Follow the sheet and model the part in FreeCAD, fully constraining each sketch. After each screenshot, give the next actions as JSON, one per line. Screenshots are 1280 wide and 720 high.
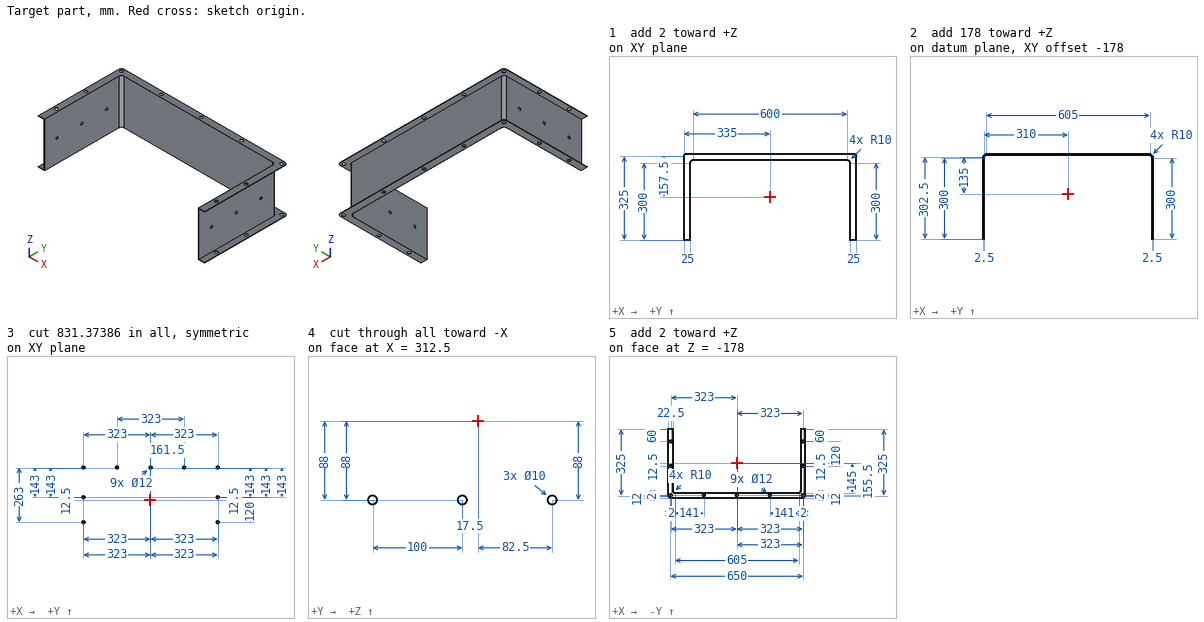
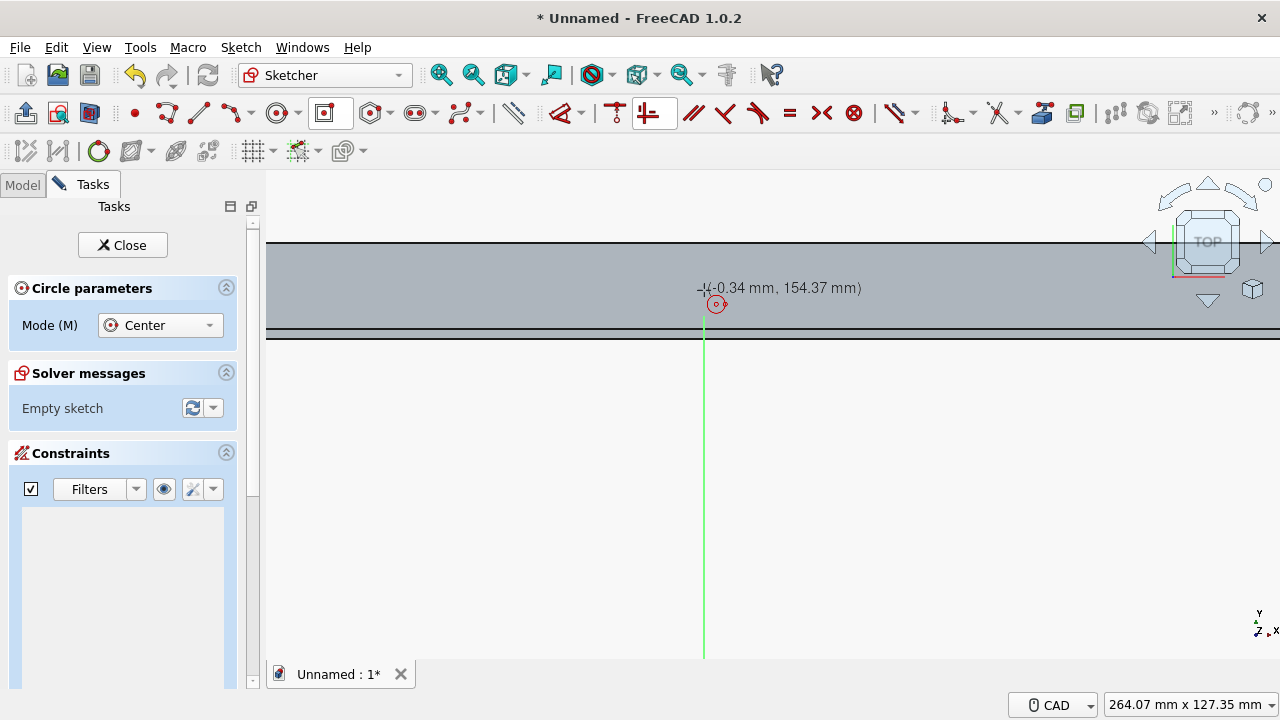
{"action": "scroll", "coordinate": [705, 290], "scroll_direction": "down", "scroll_amount": 7}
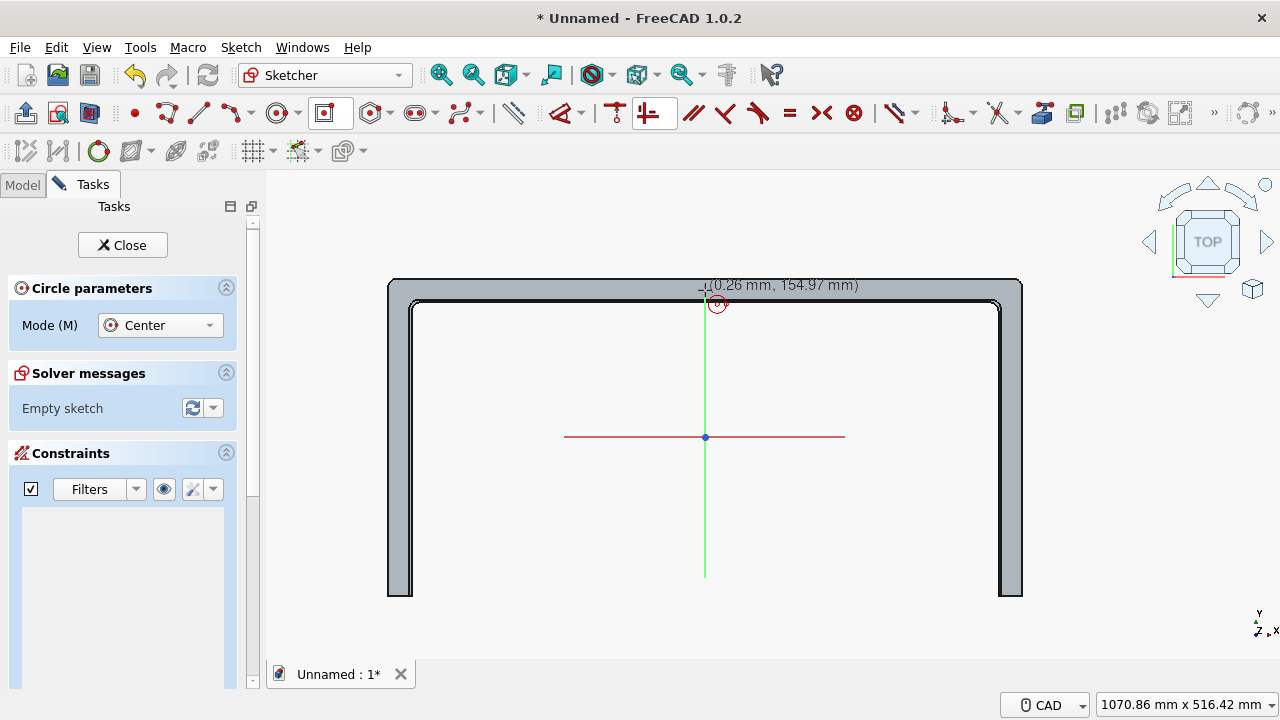
{"action": "left_click", "coordinate": [705, 290]}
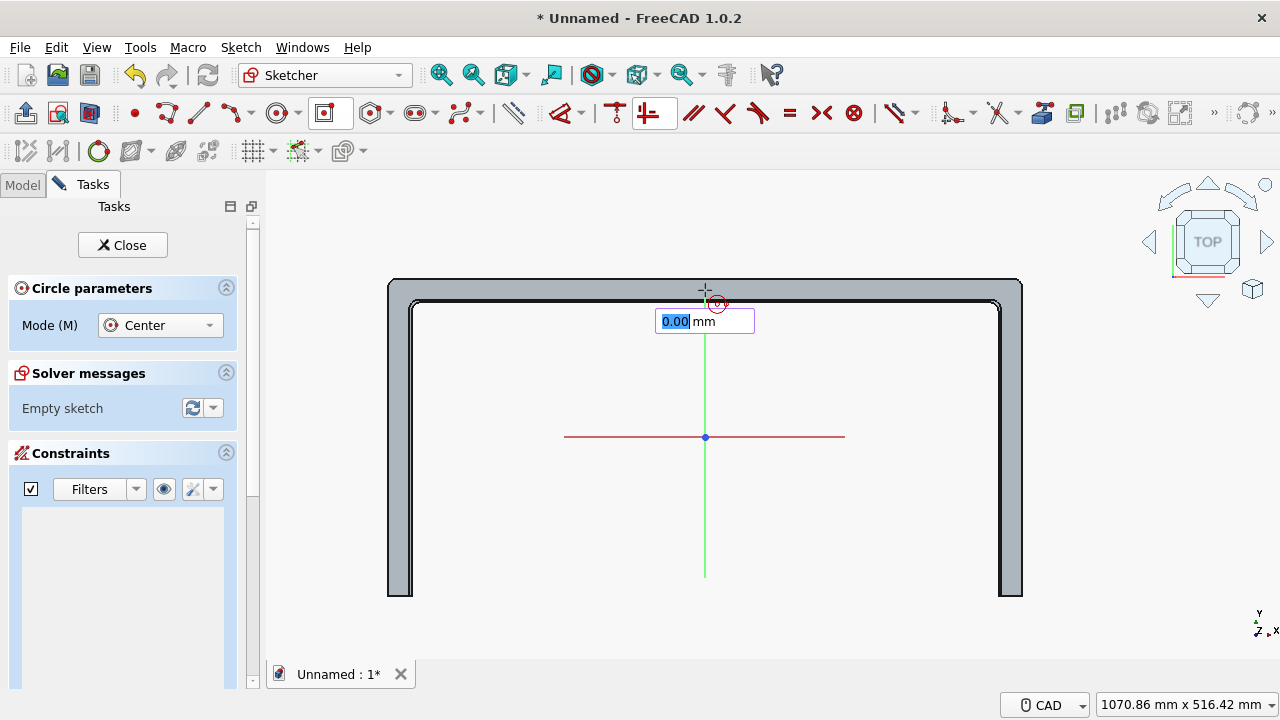
{"action": "scroll", "coordinate": [710, 288], "scroll_direction": "up", "scroll_amount": 6}
{"action": "mouse_move", "coordinate": [710, 287]}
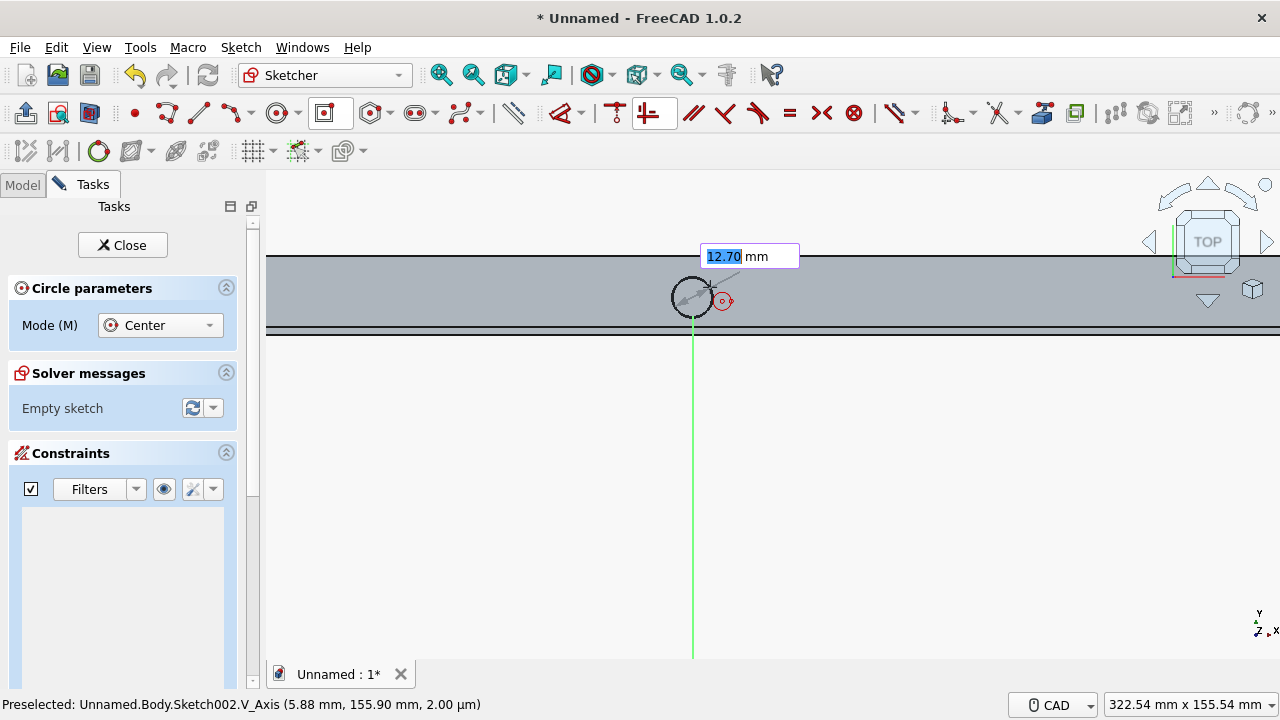
{"action": "type", "text": "12"}
{"action": "key", "text": "Return"}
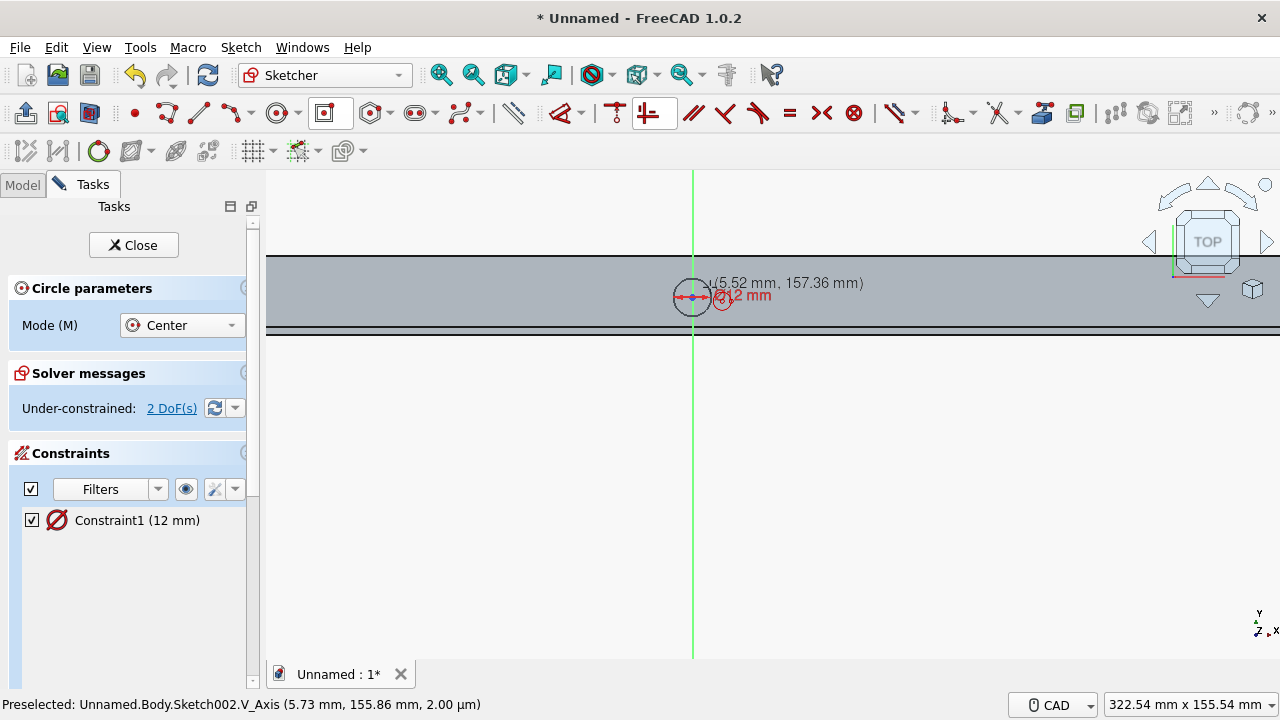
{"action": "scroll", "coordinate": [710, 288], "scroll_direction": "down", "scroll_amount": 6}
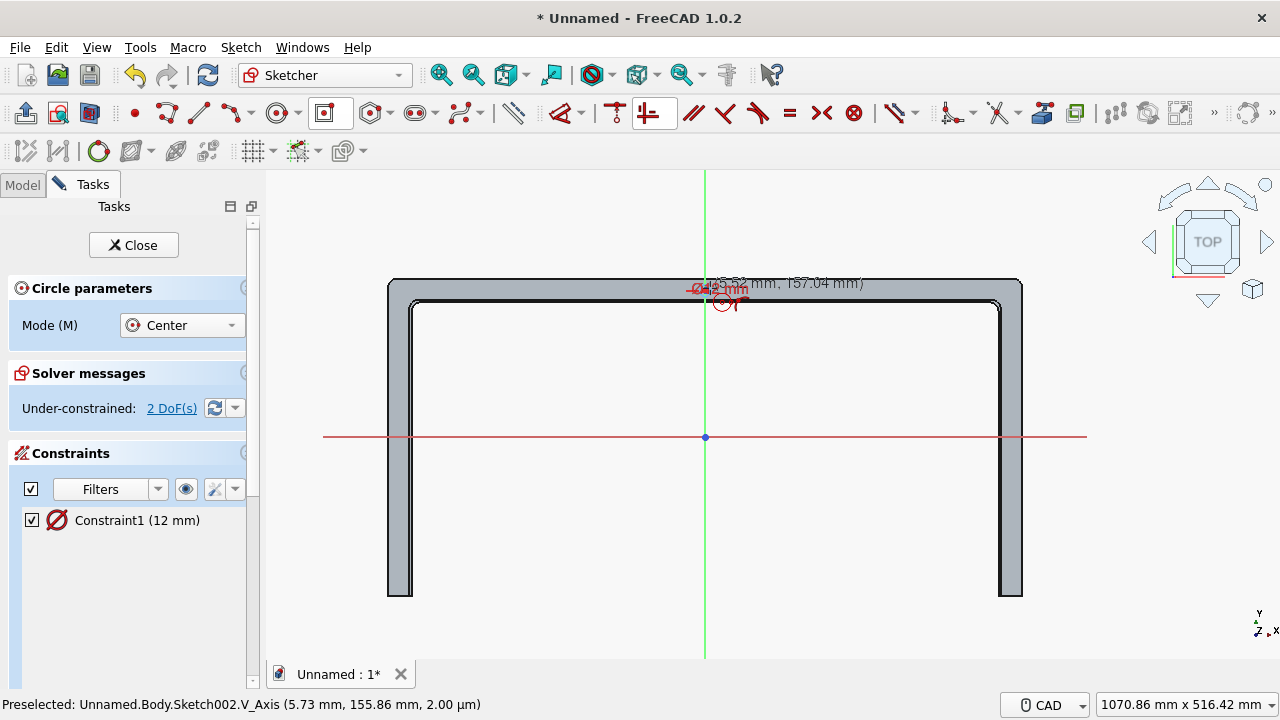
{"action": "scroll", "coordinate": [858, 290], "scroll_direction": "up", "scroll_amount": 7}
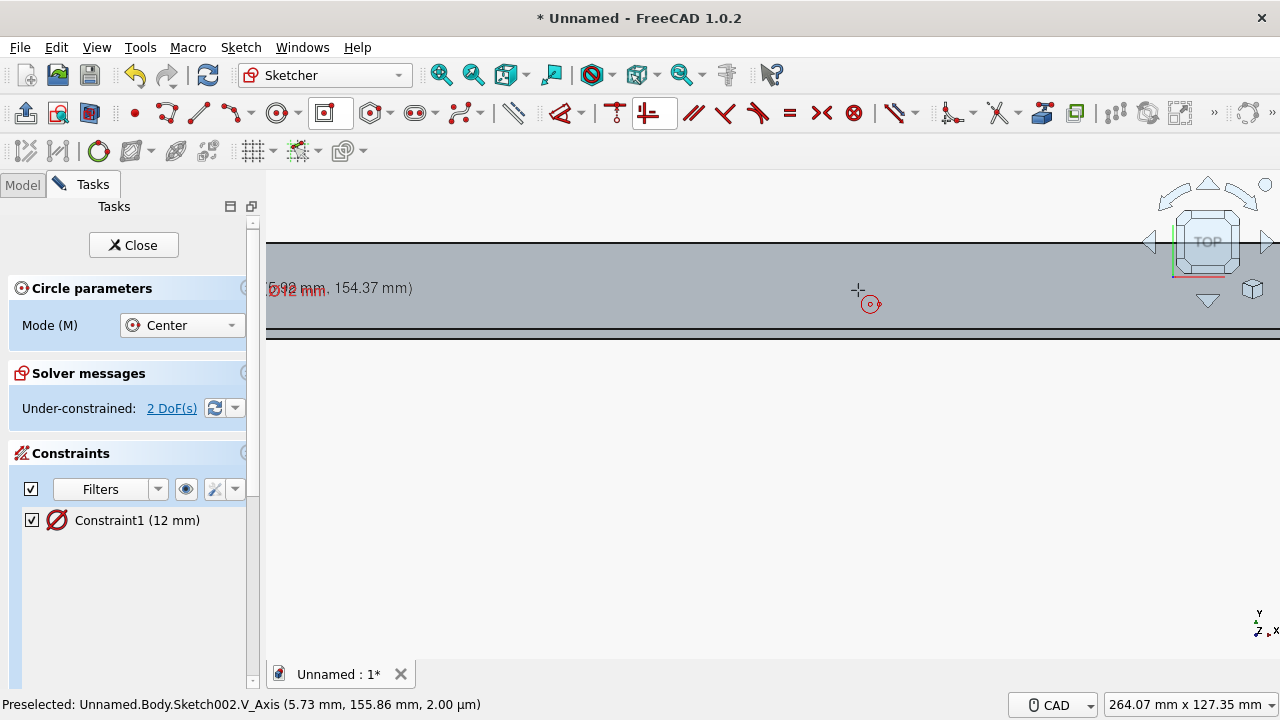
{"action": "scroll", "coordinate": [858, 290], "scroll_direction": "down", "scroll_amount": 7}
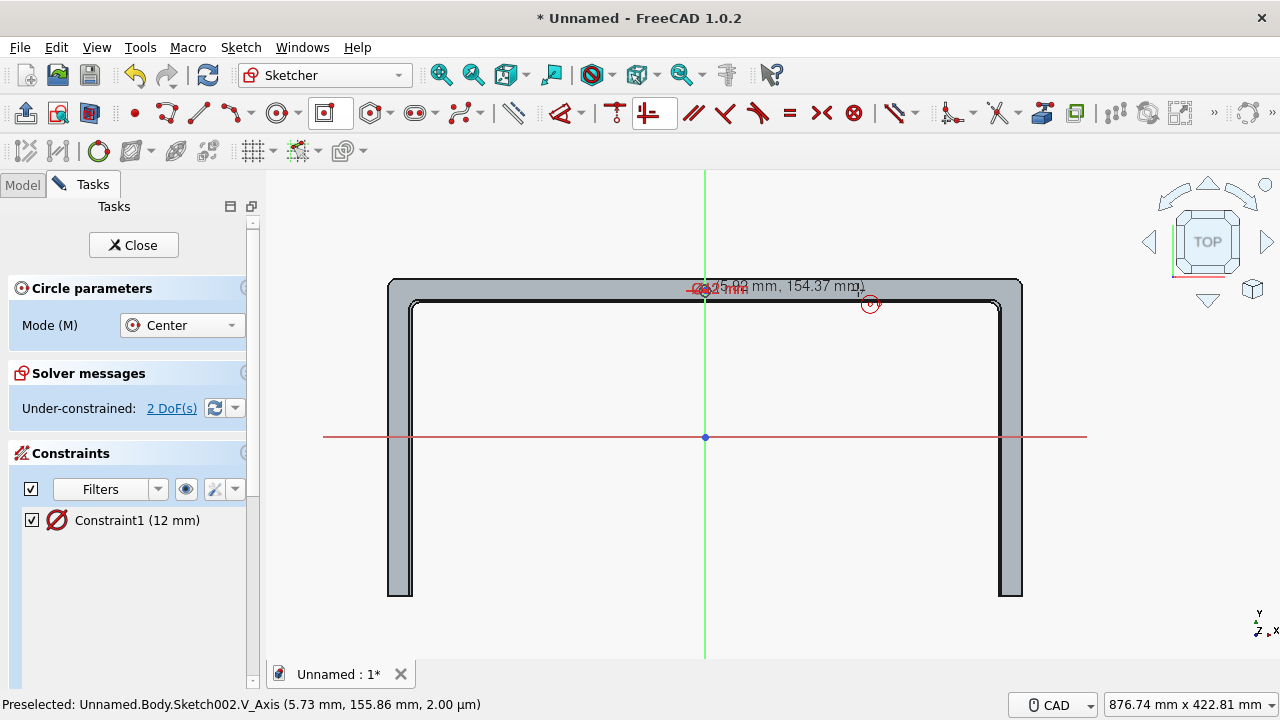
{"action": "left_click", "coordinate": [858, 290]}
{"action": "mouse_move", "coordinate": [862, 286]}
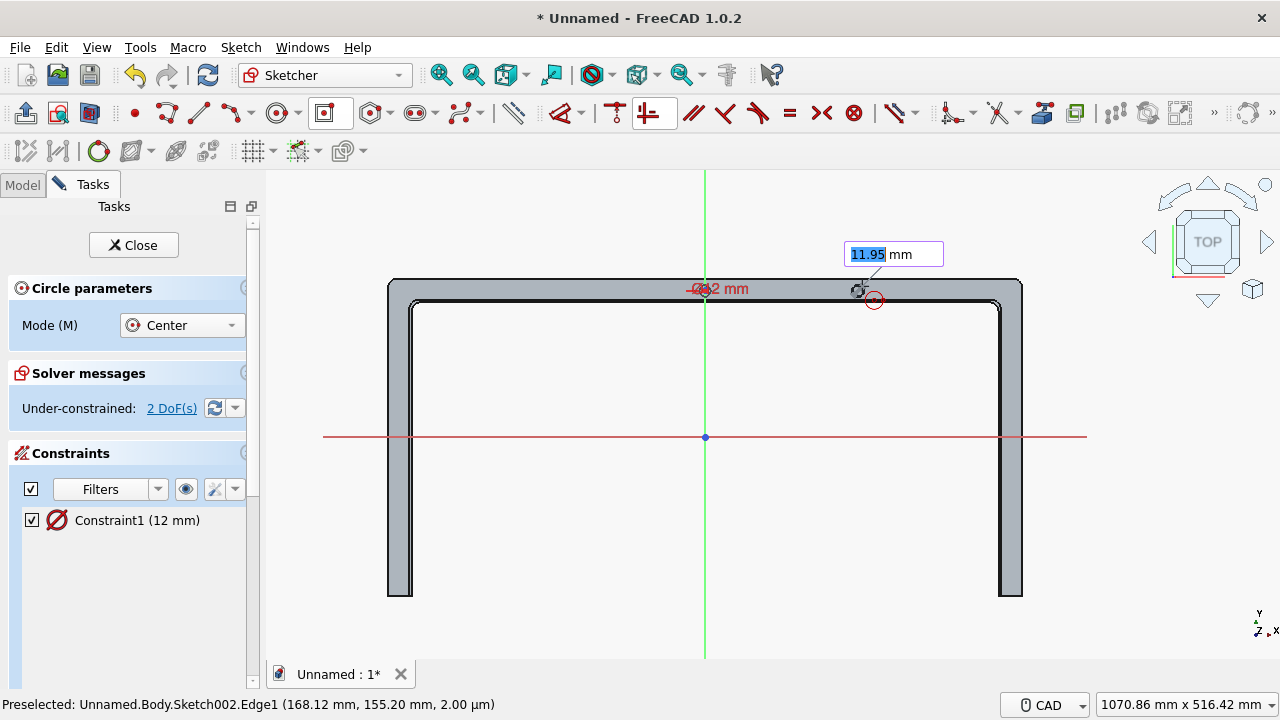
{"action": "type", "text": "12"}
{"action": "key", "text": "Return"}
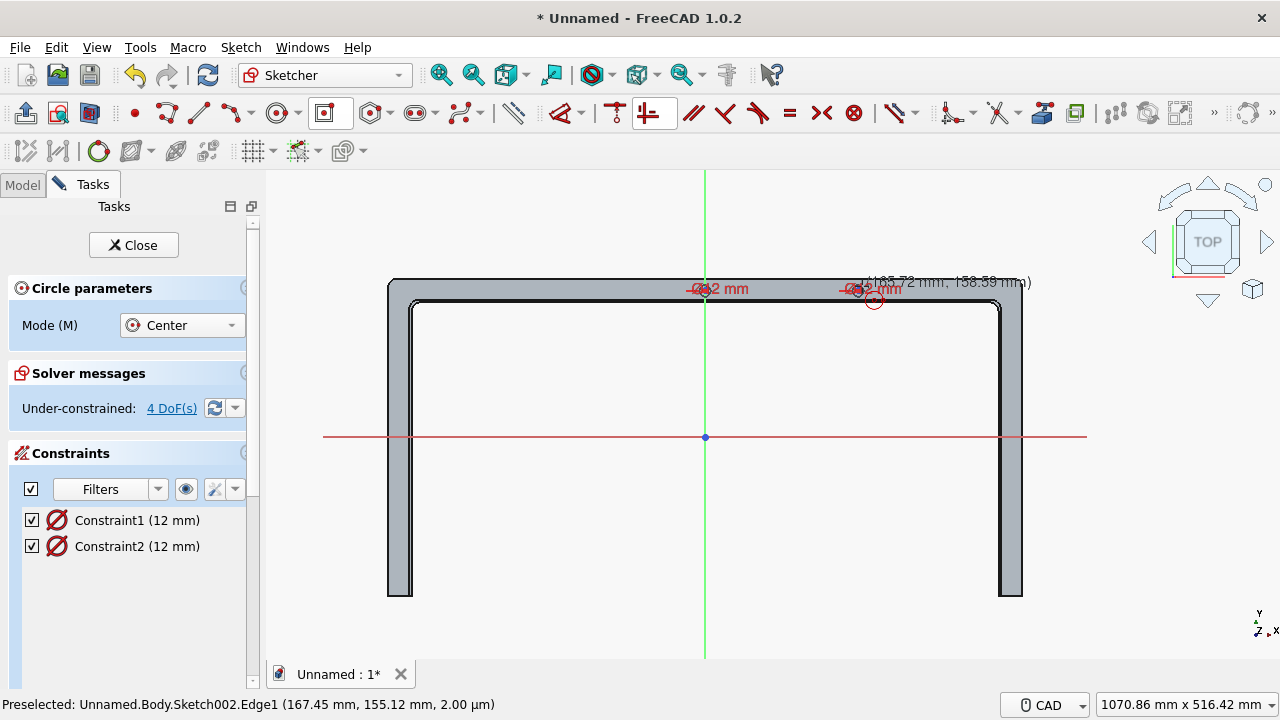
{"action": "scroll", "coordinate": [1011, 425], "scroll_direction": "up", "scroll_amount": 7}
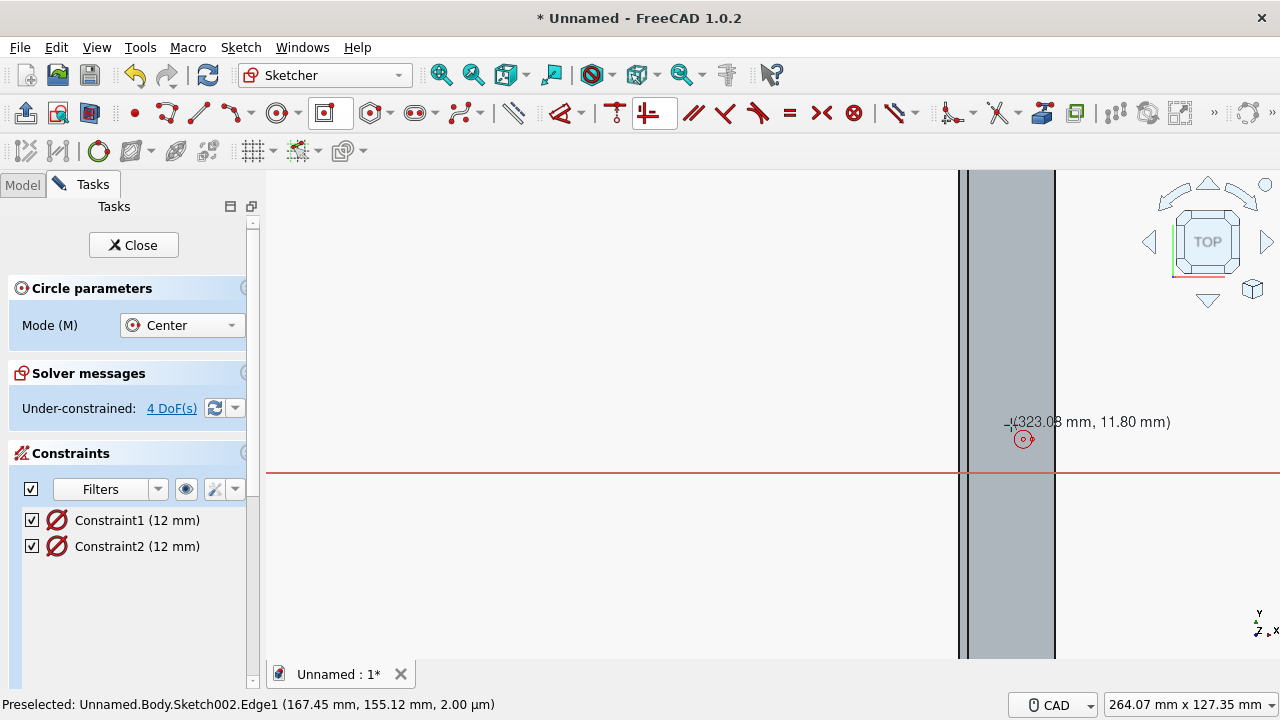
{"action": "scroll", "coordinate": [1011, 426], "scroll_direction": "down", "scroll_amount": 7}